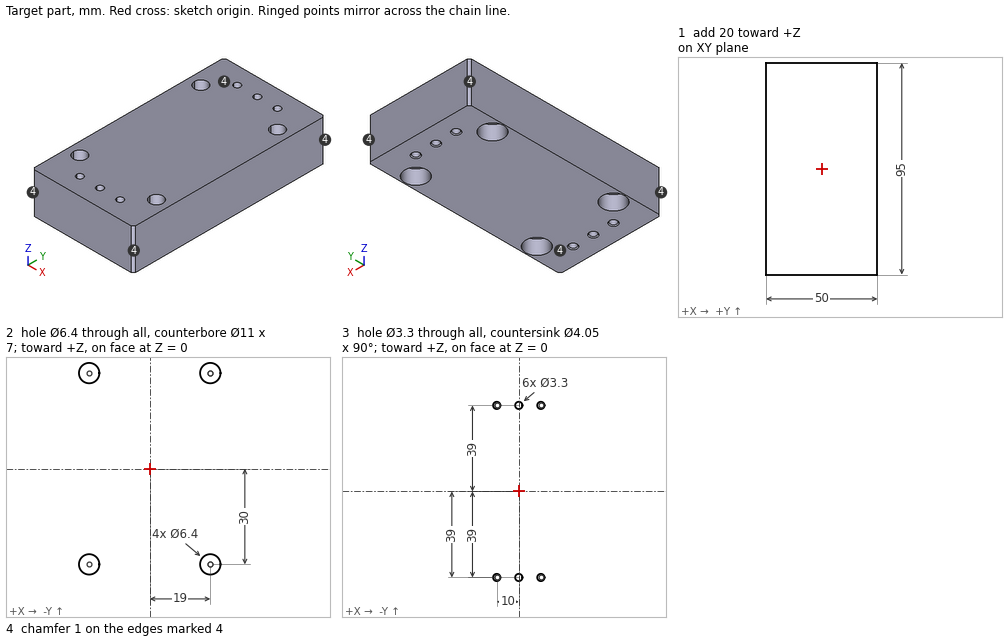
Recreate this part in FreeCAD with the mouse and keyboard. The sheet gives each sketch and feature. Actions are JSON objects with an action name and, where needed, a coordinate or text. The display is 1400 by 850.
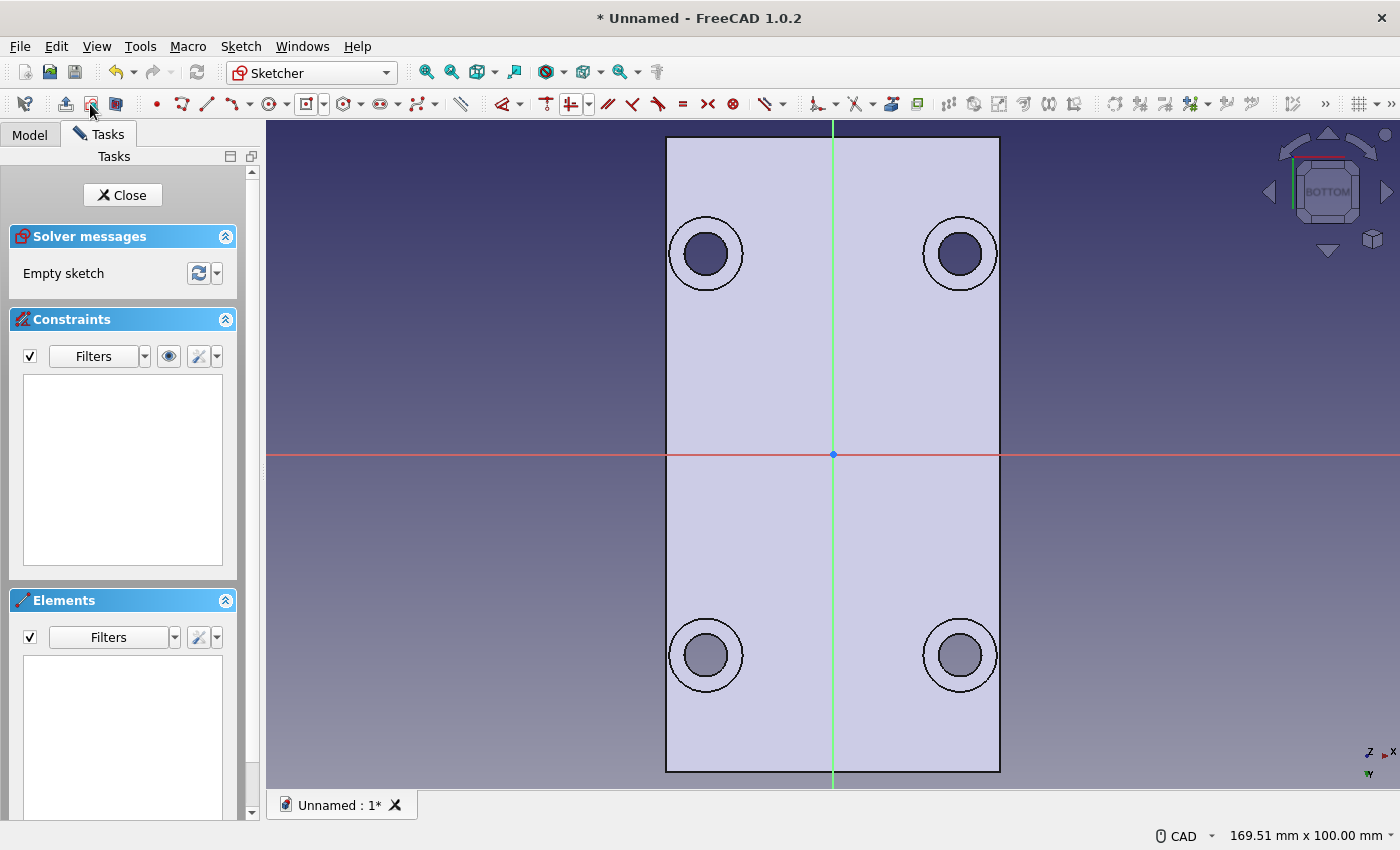
{"action": "left_click", "coordinate": [268, 104]}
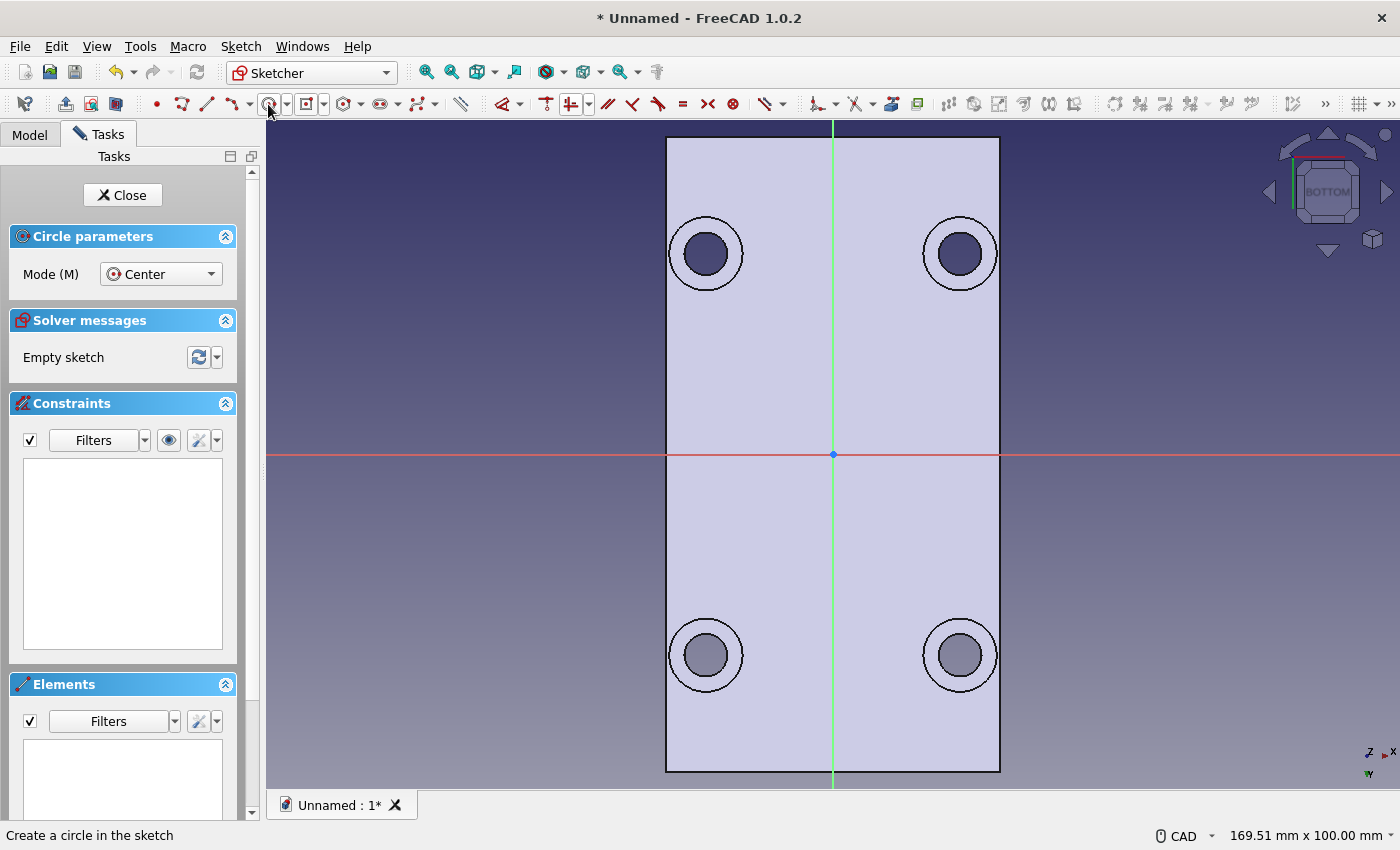
{"action": "scroll", "coordinate": [833, 194], "scroll_direction": "up", "scroll_amount": 4}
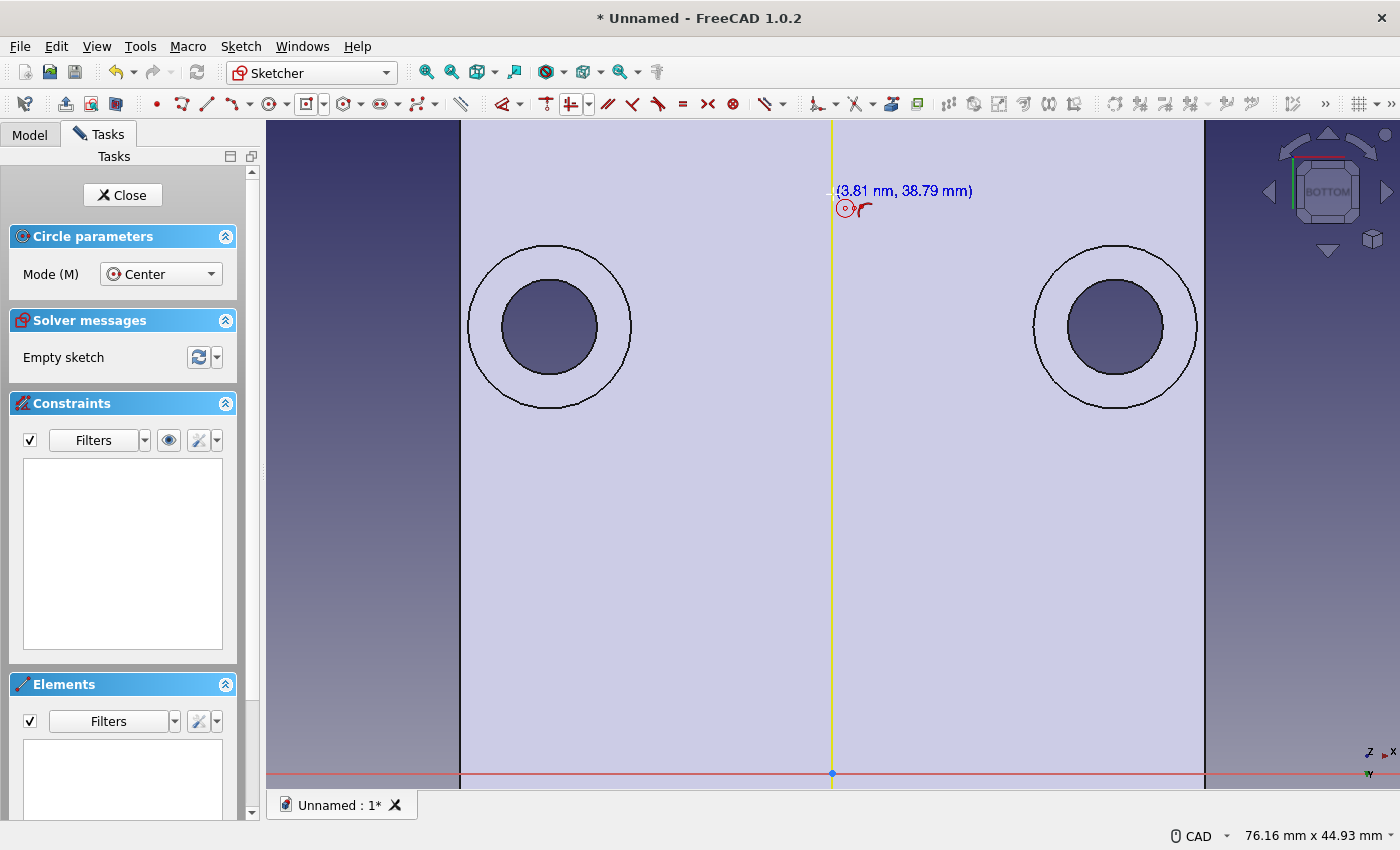
{"action": "left_click", "coordinate": [832, 193]}
{"action": "left_click", "coordinate": [850, 176]}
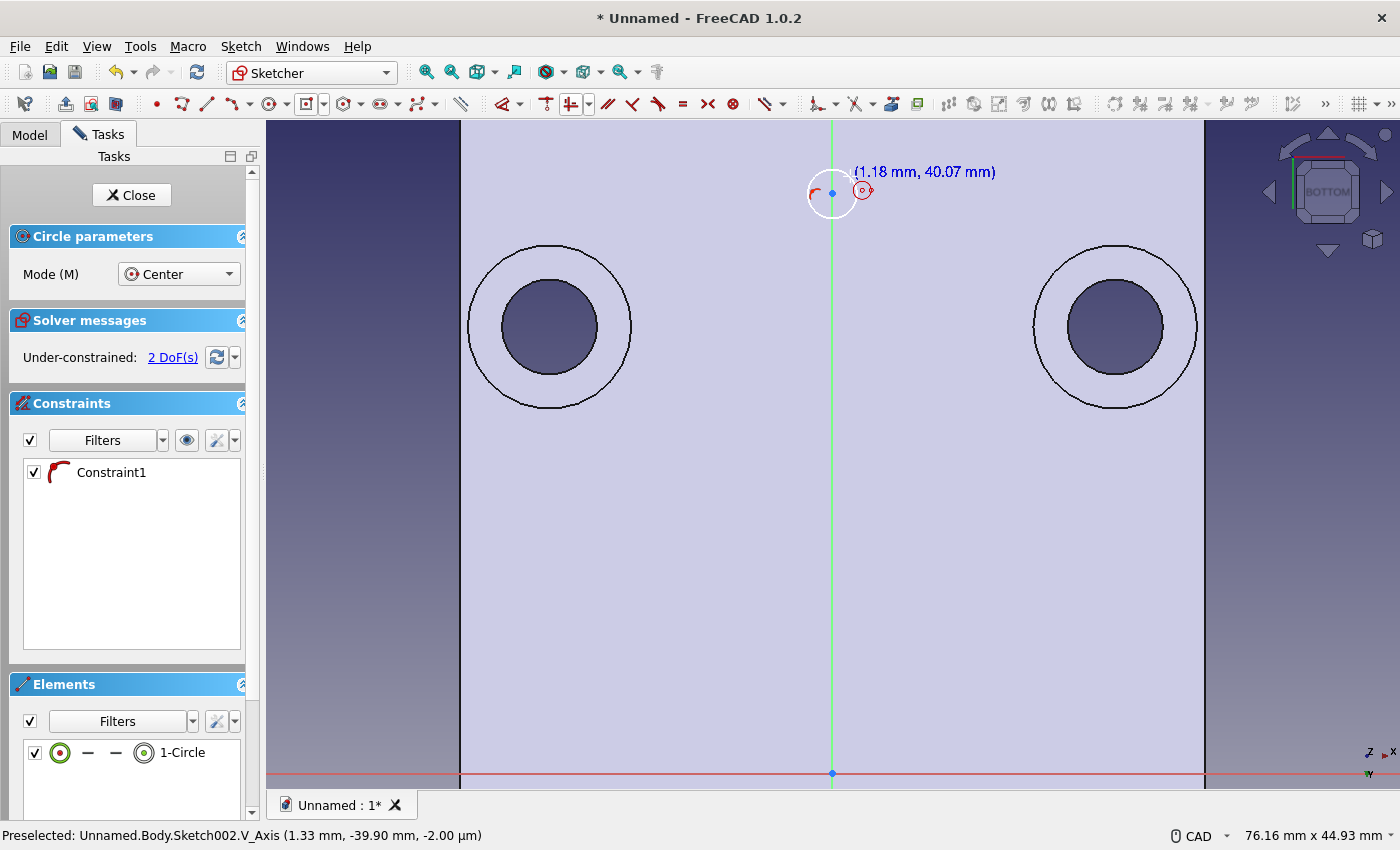
{"action": "scroll", "coordinate": [725, 269], "scroll_direction": "down", "scroll_amount": 5}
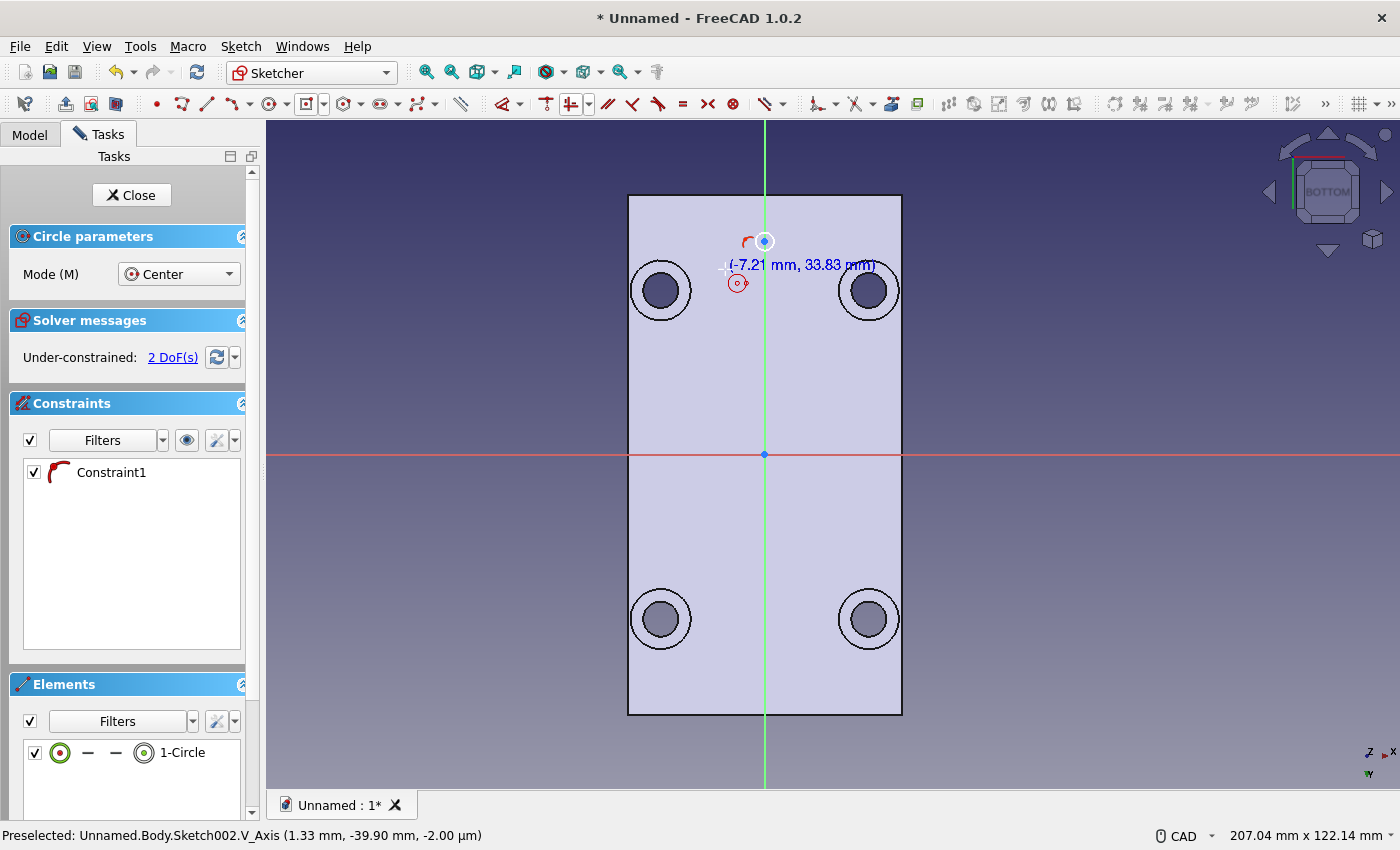
{"action": "scroll", "coordinate": [710, 668], "scroll_direction": "up", "scroll_amount": 5}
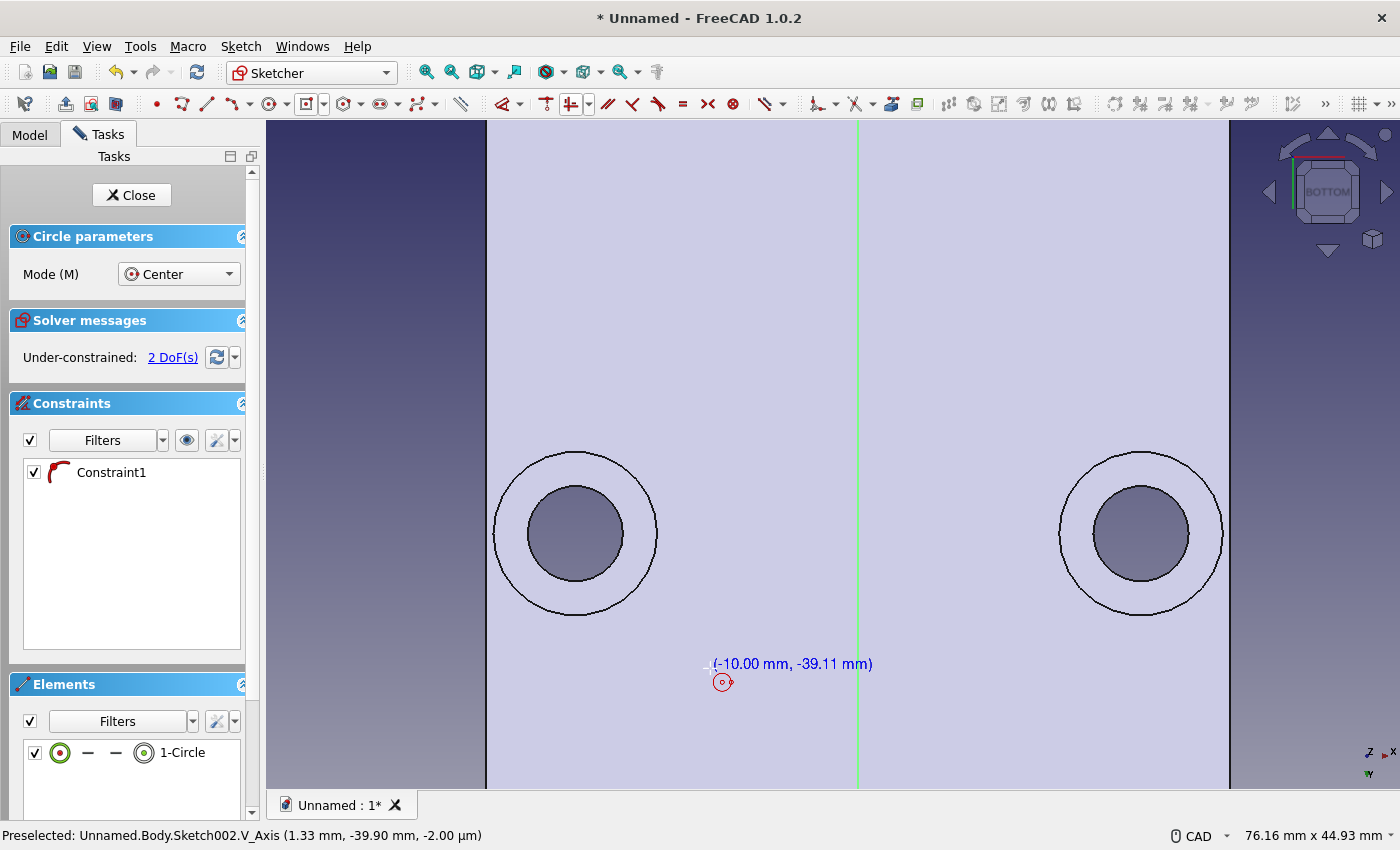
{"action": "left_click", "coordinate": [709, 668]}
{"action": "left_click", "coordinate": [727, 650]}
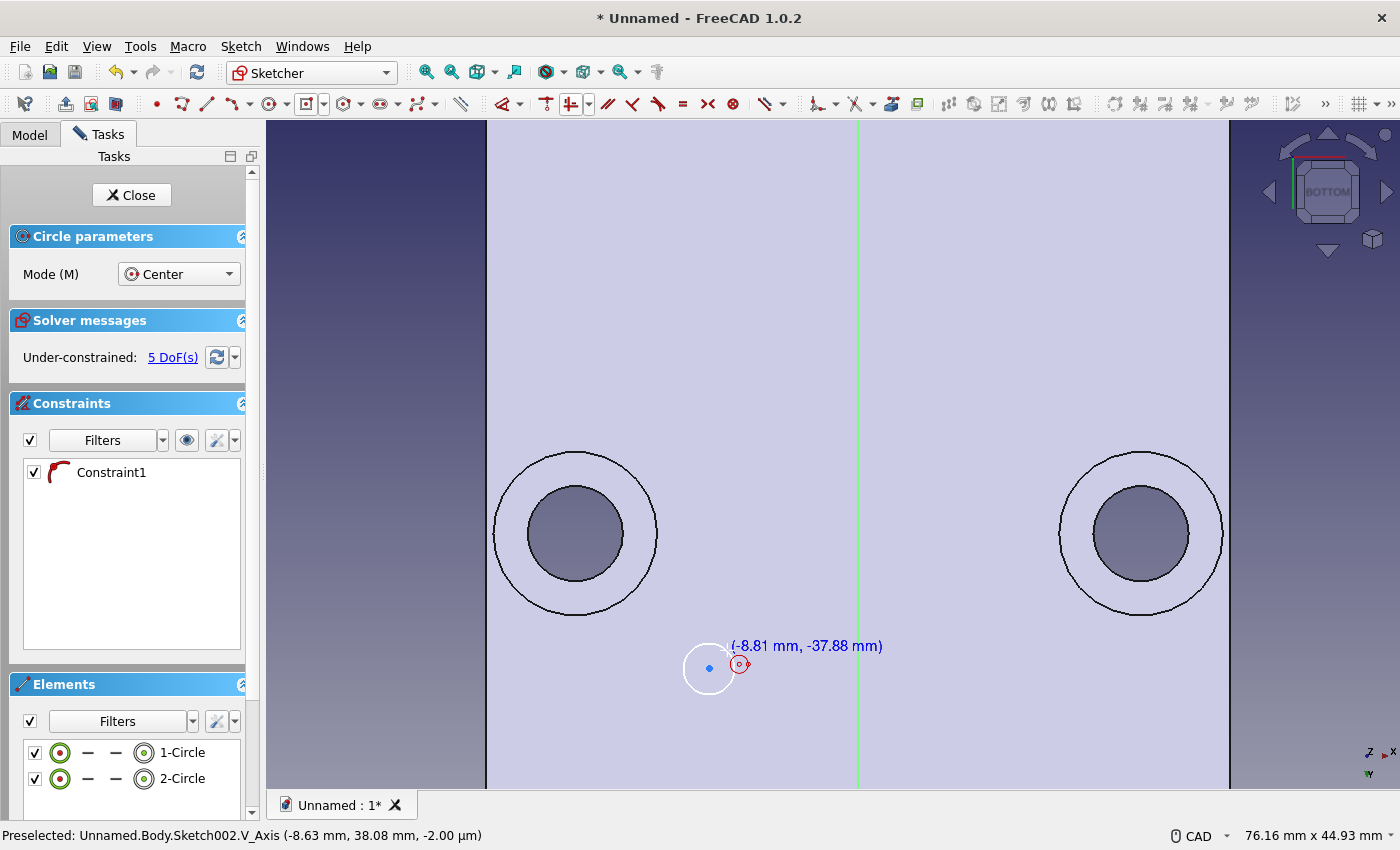
{"action": "scroll", "coordinate": [710, 668], "scroll_direction": "down", "scroll_amount": 5}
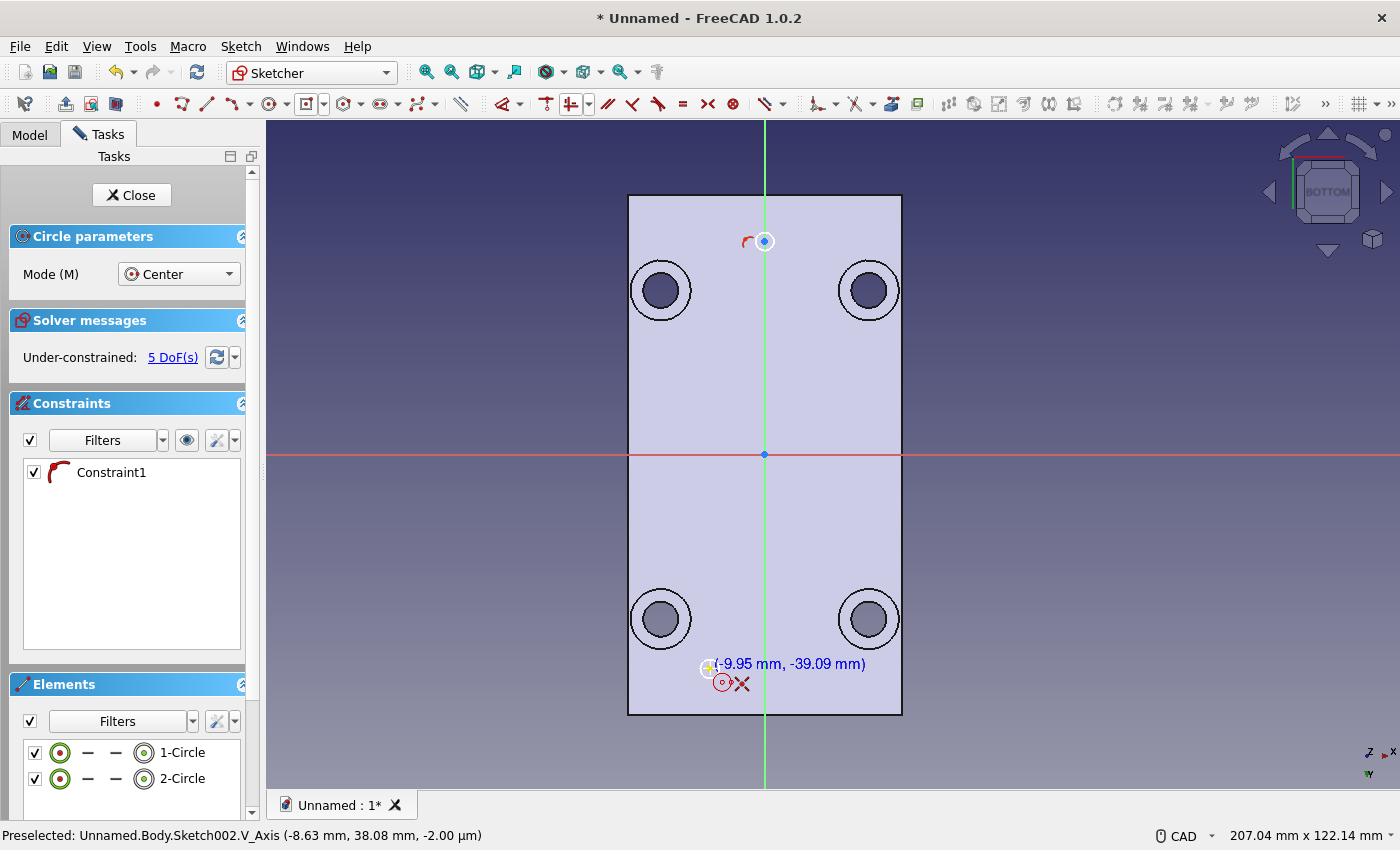
{"action": "scroll", "coordinate": [710, 241], "scroll_direction": "up", "scroll_amount": 5}